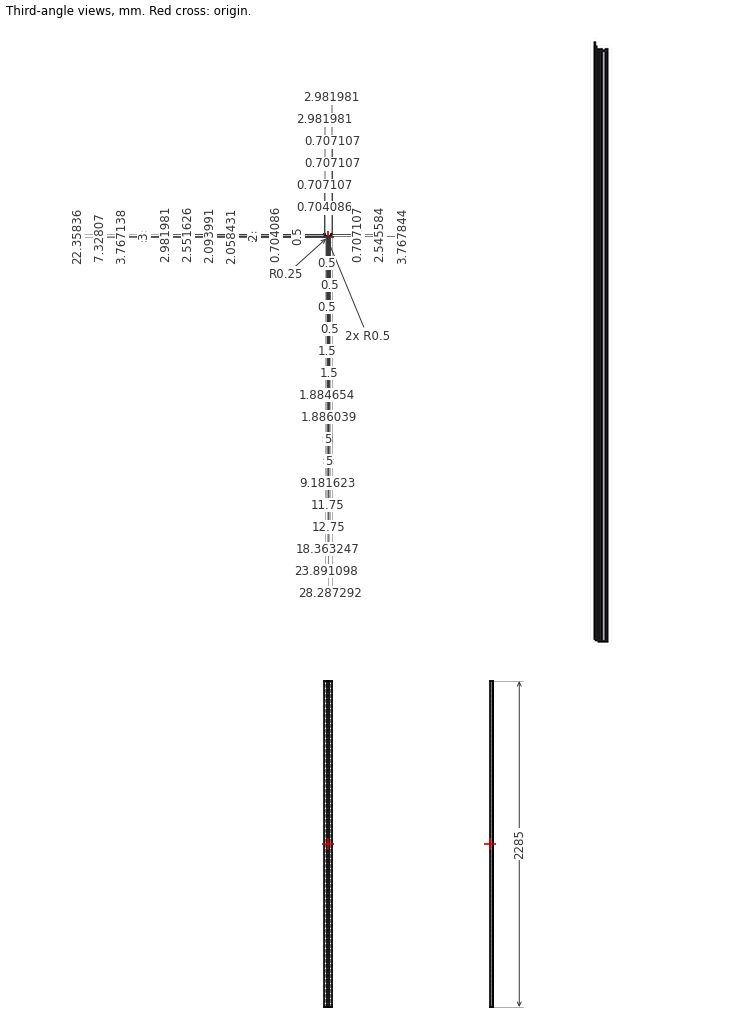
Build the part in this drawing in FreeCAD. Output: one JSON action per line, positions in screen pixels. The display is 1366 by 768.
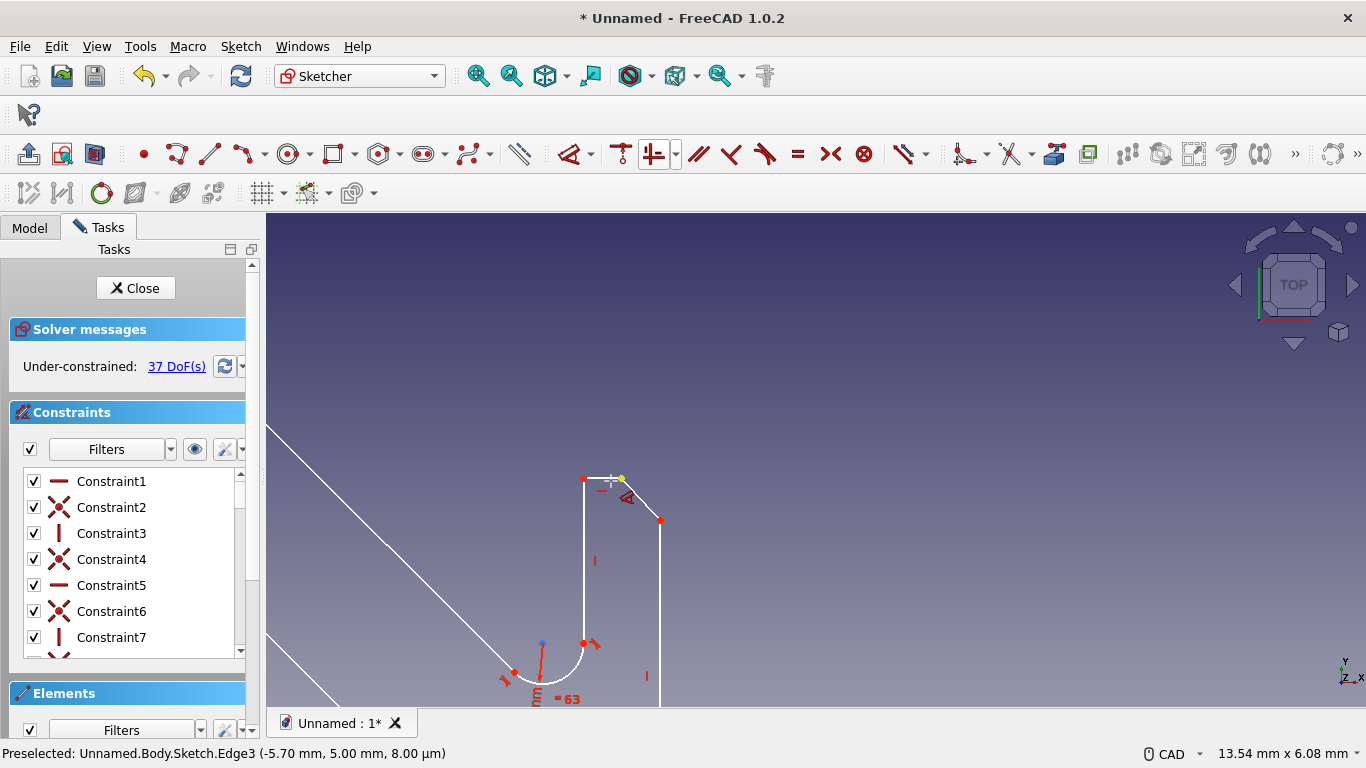
{"action": "left_click", "coordinate": [606, 478]}
{"action": "left_click", "coordinate": [602, 512]}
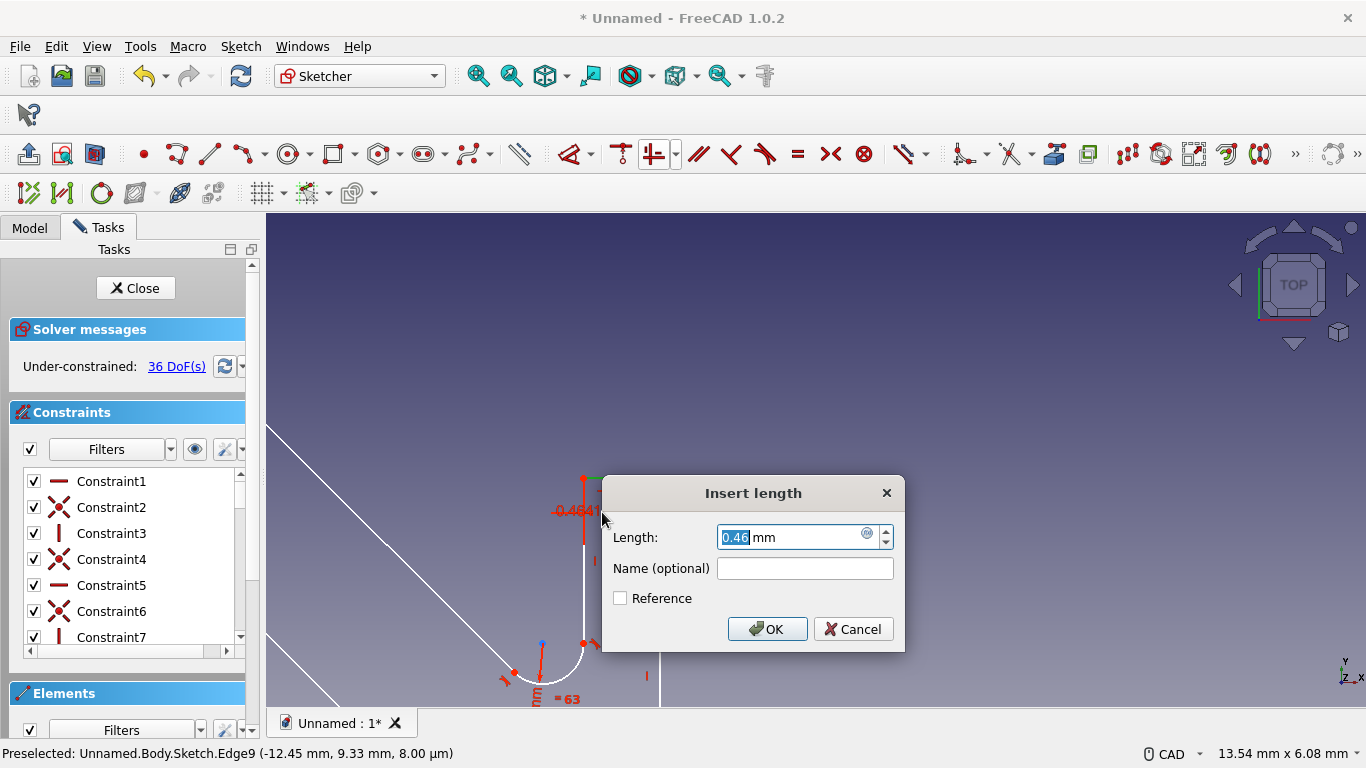
{"action": "type", "text": "0.5"}
{"action": "key", "text": "Return"}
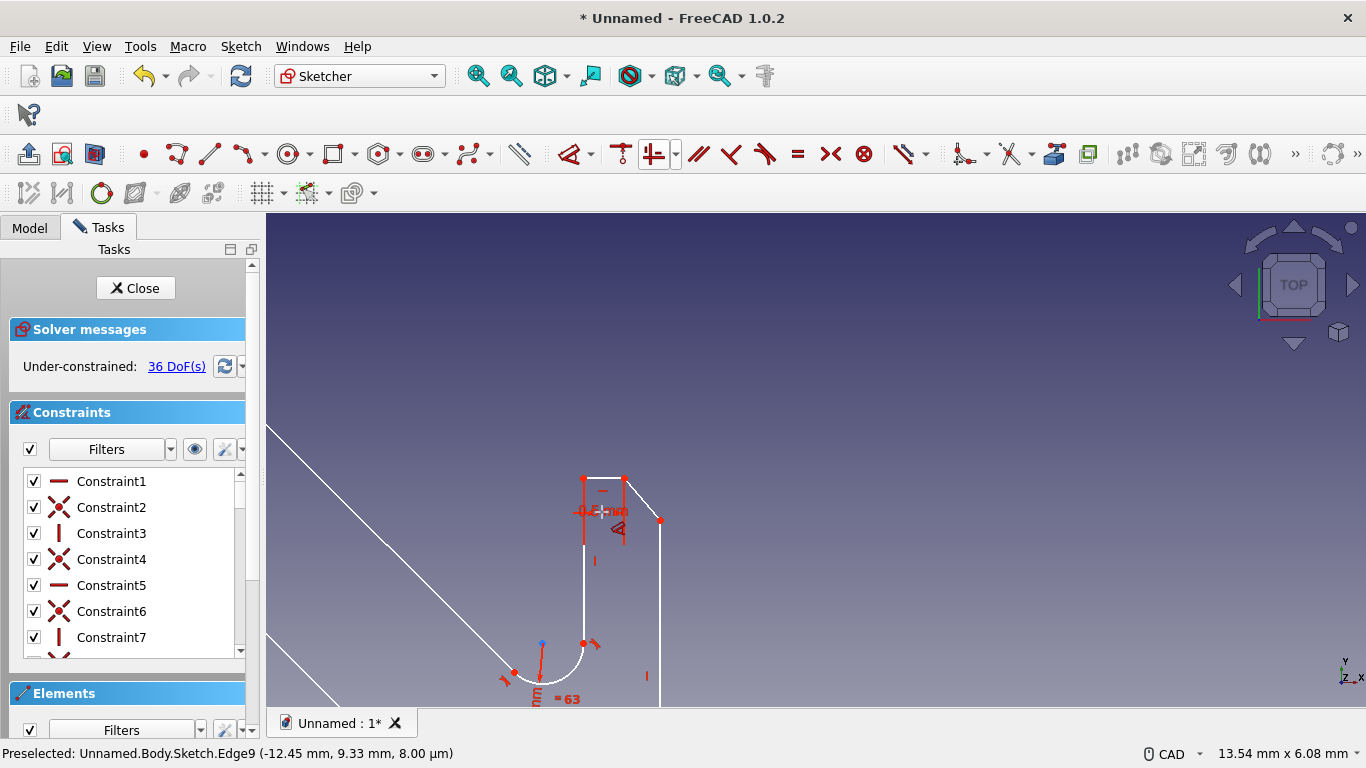
{"action": "scroll", "coordinate": [611, 481], "scroll_direction": "down", "scroll_amount": 10}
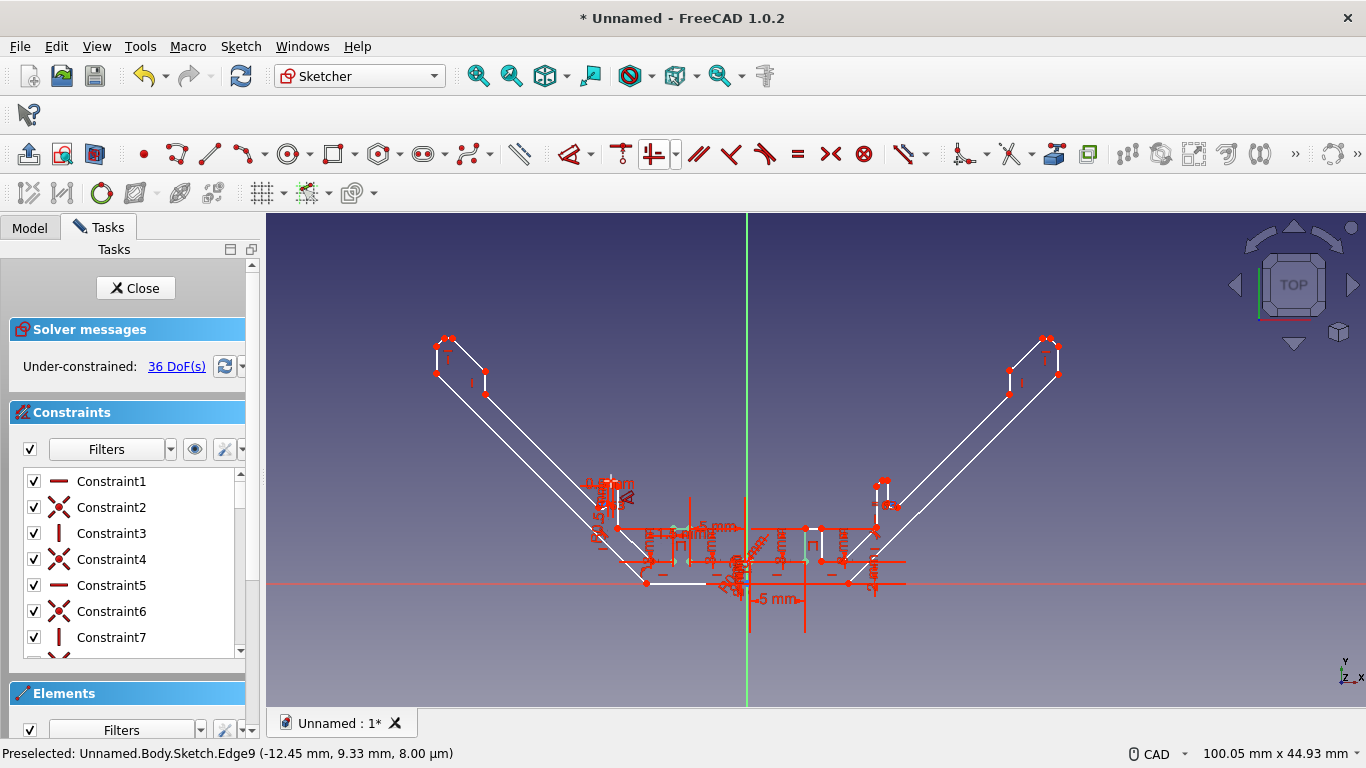
{"action": "scroll", "coordinate": [886, 481], "scroll_direction": "up", "scroll_amount": 11}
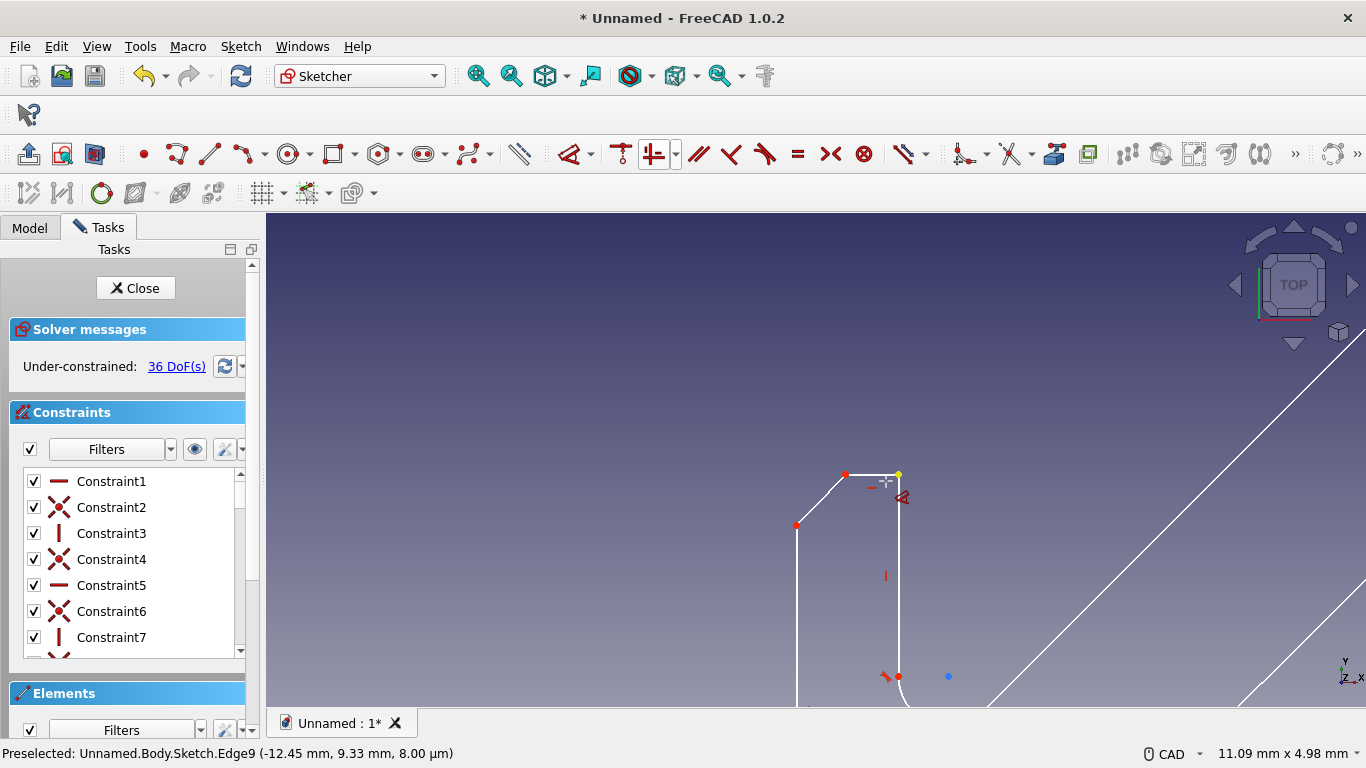
{"action": "left_click", "coordinate": [883, 475]}
{"action": "left_click", "coordinate": [872, 509]}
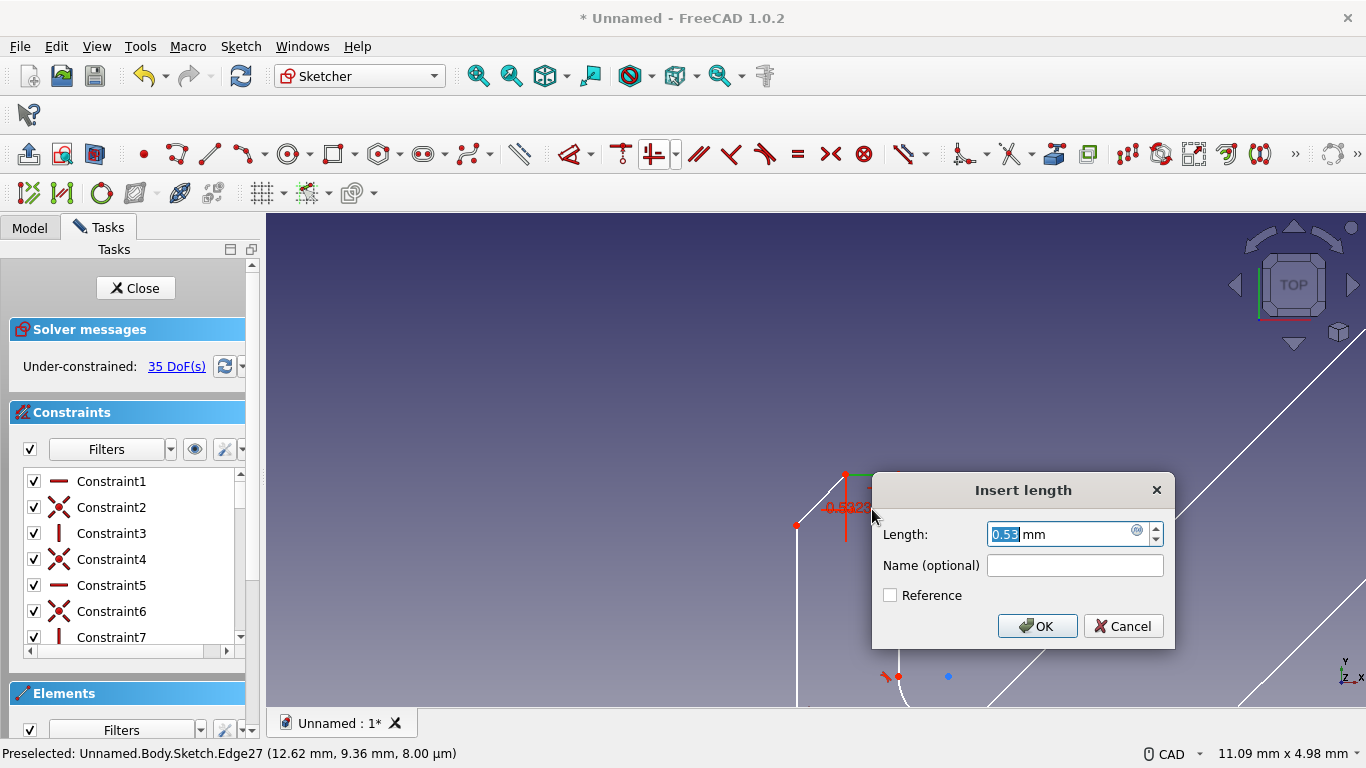
{"action": "type", "text": "0.5"}
{"action": "key", "text": "Return"}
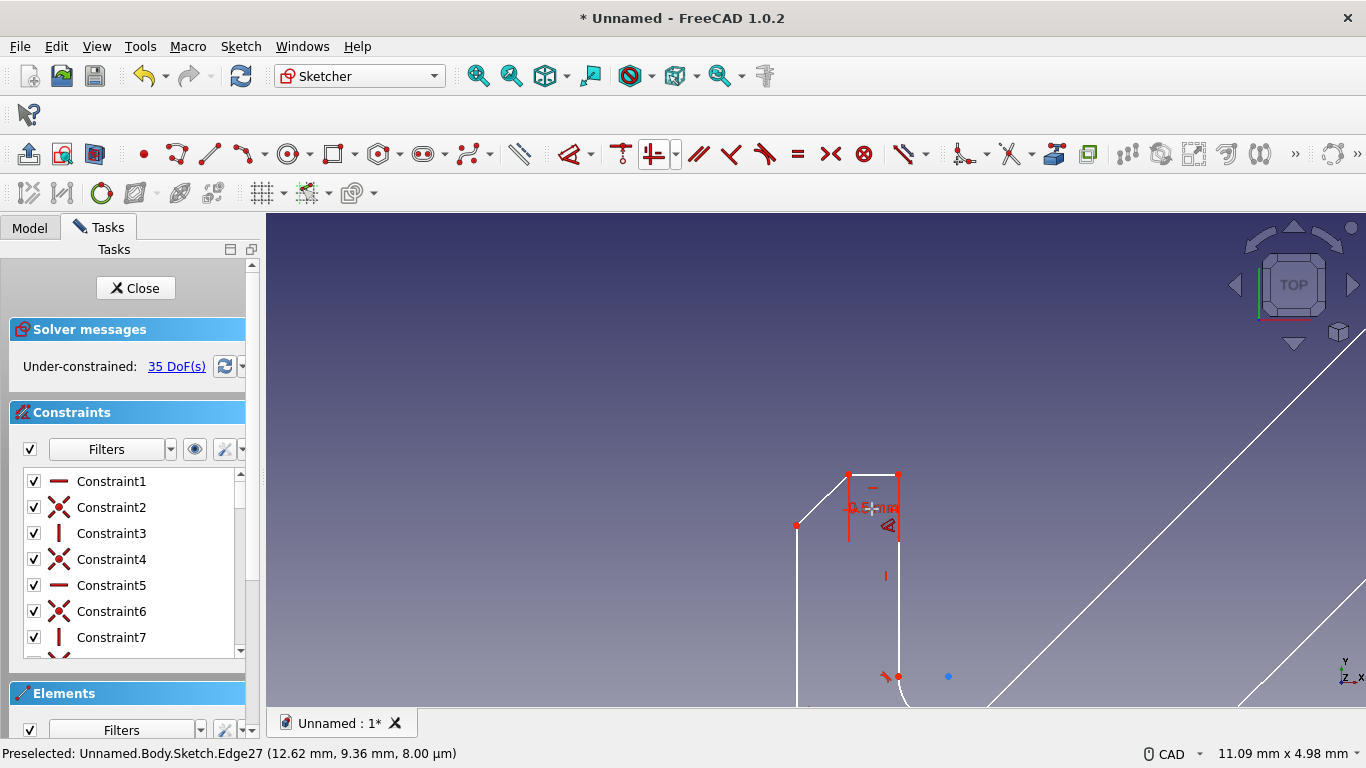
{"action": "scroll", "coordinate": [887, 481], "scroll_direction": "down", "scroll_amount": 11}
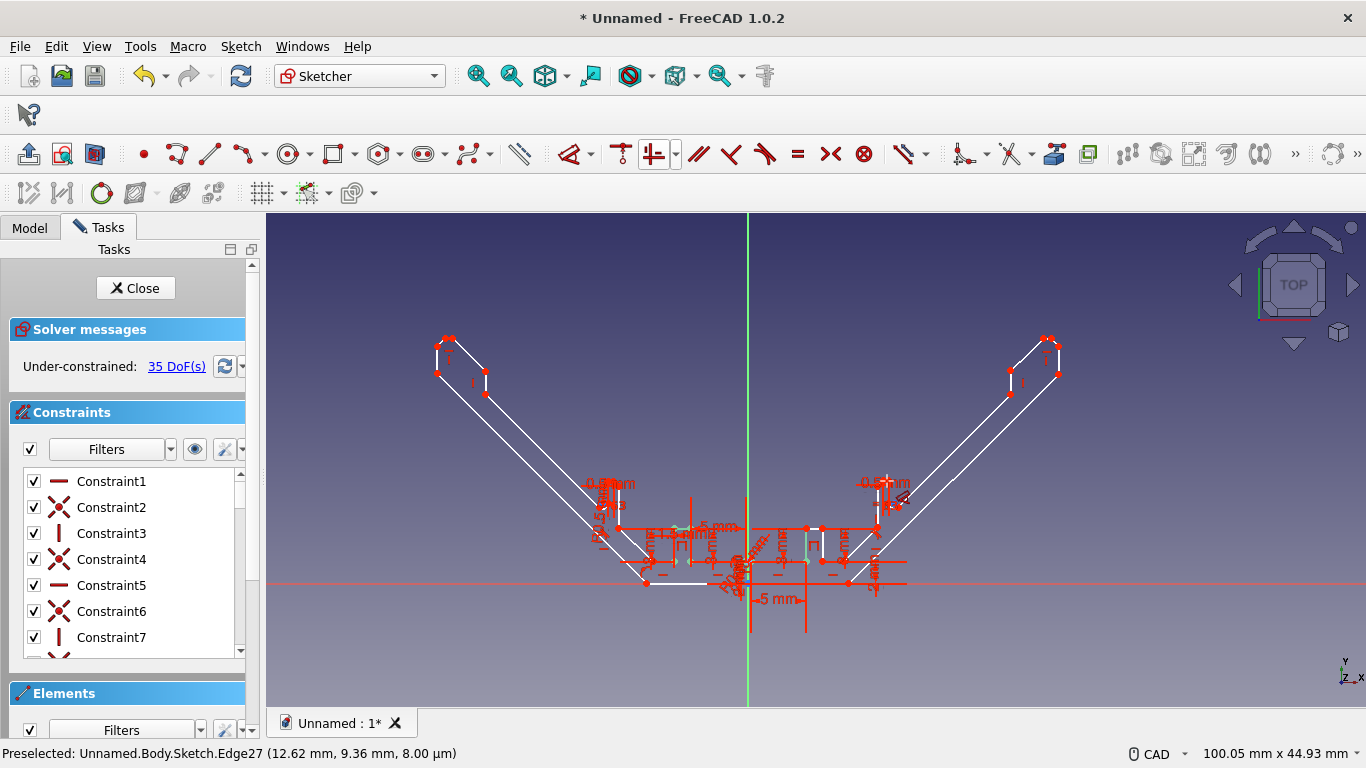
{"action": "scroll", "coordinate": [818, 529], "scroll_direction": "up", "scroll_amount": 6}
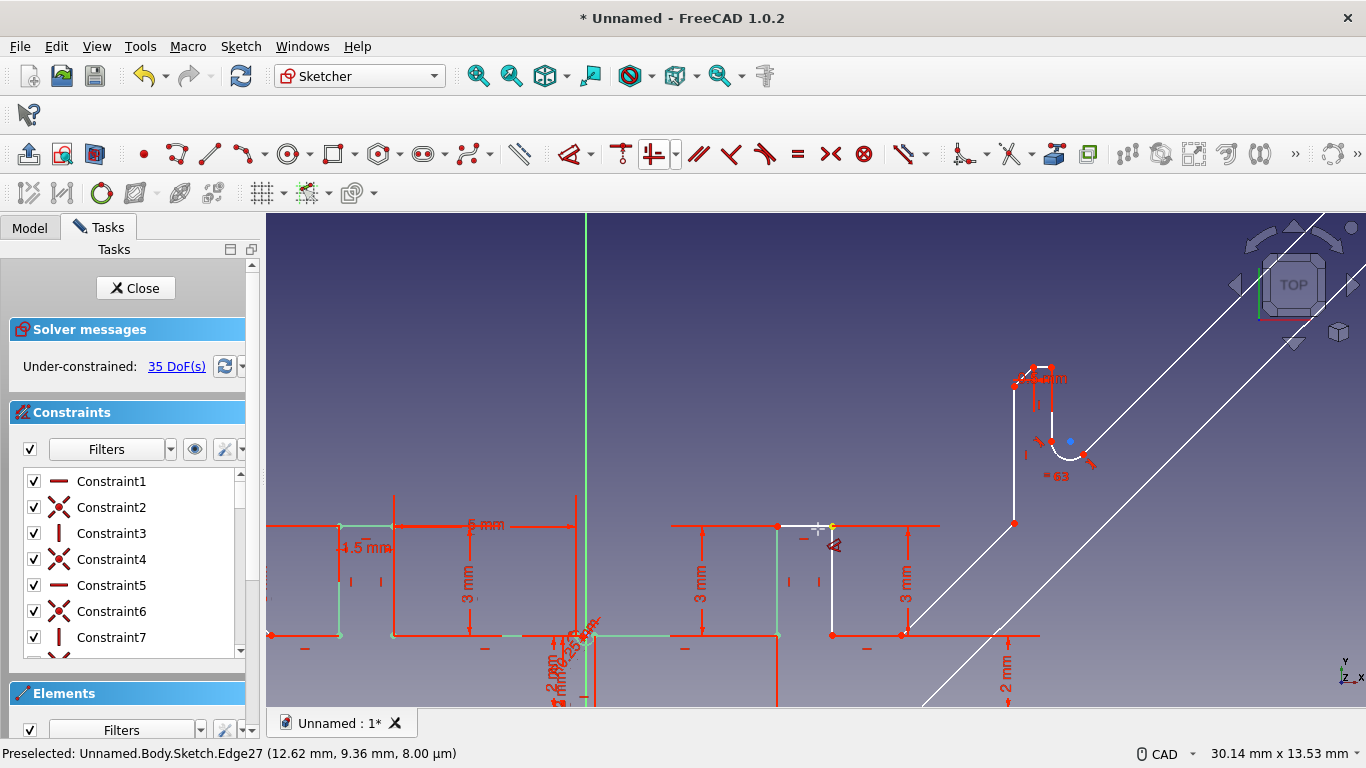
{"action": "left_click", "coordinate": [816, 526]}
{"action": "left_click", "coordinate": [805, 560]}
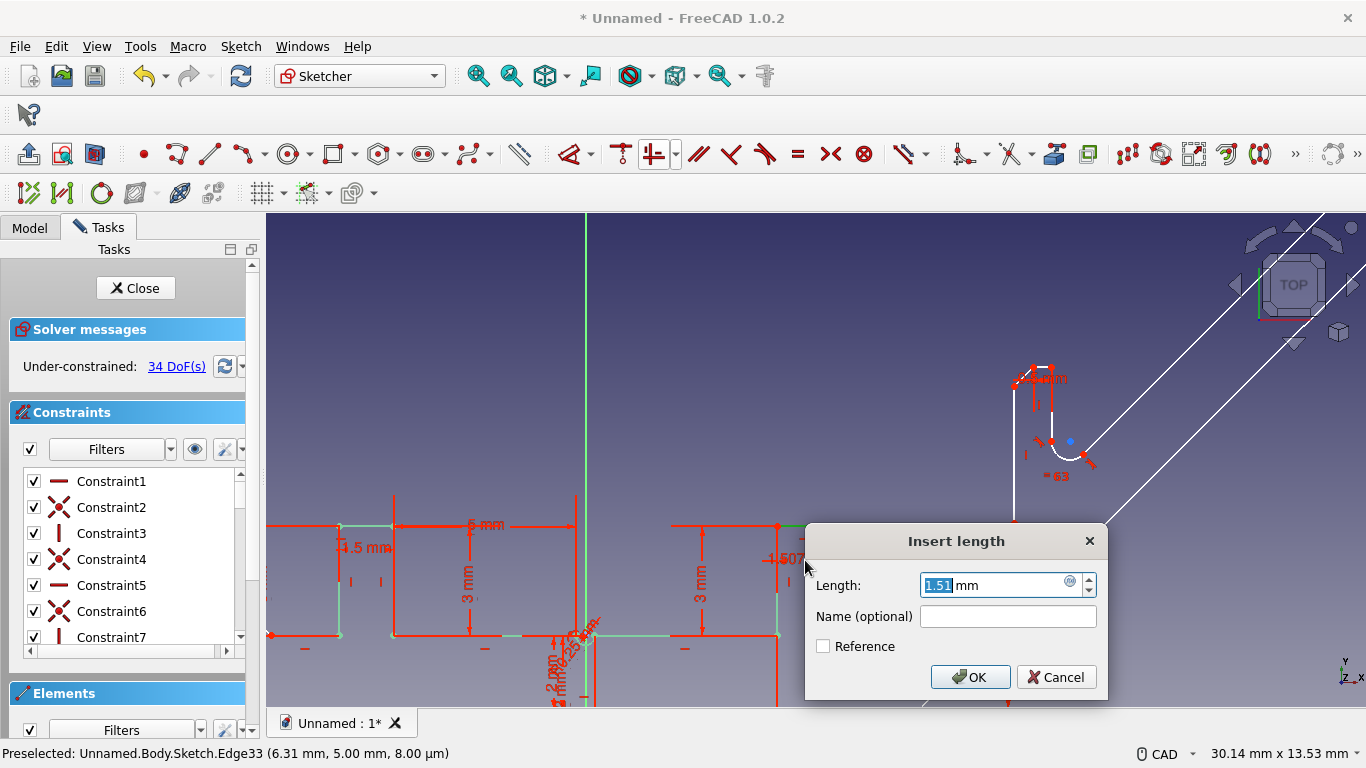
{"action": "type", "text": "1.5"}
{"action": "key", "text": "Return"}